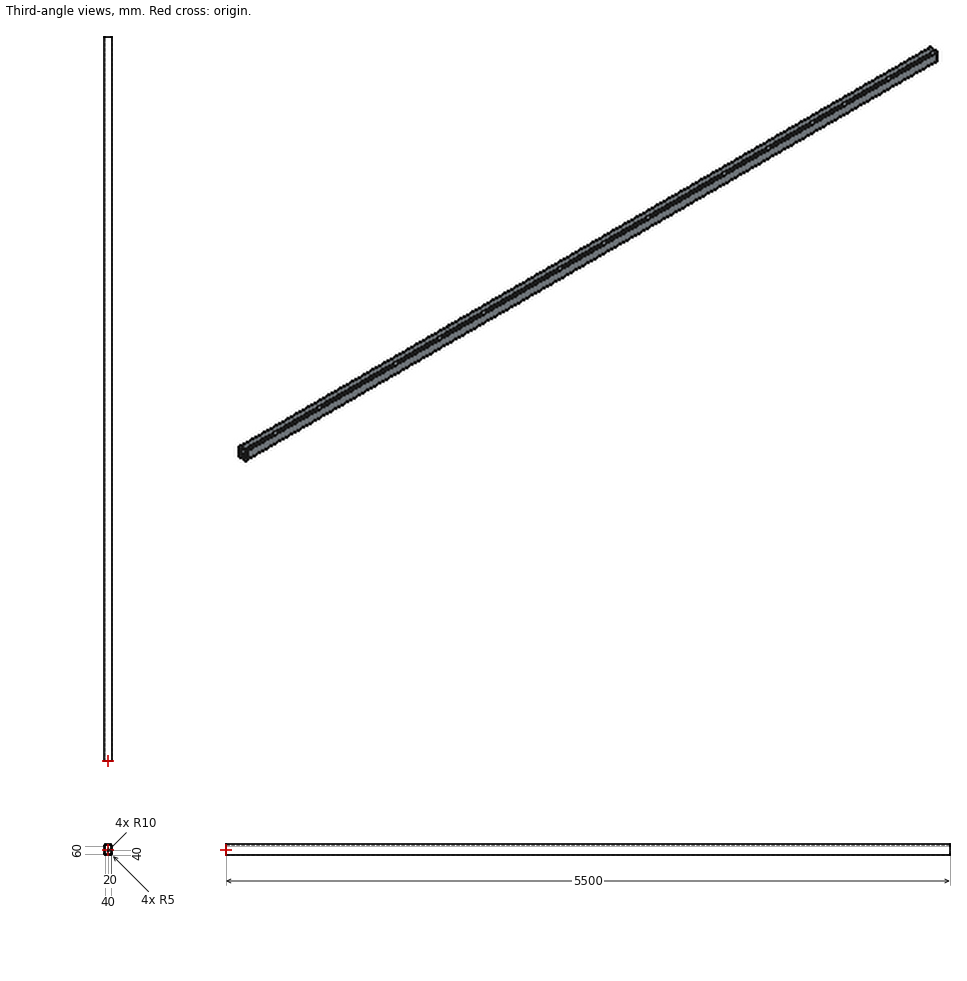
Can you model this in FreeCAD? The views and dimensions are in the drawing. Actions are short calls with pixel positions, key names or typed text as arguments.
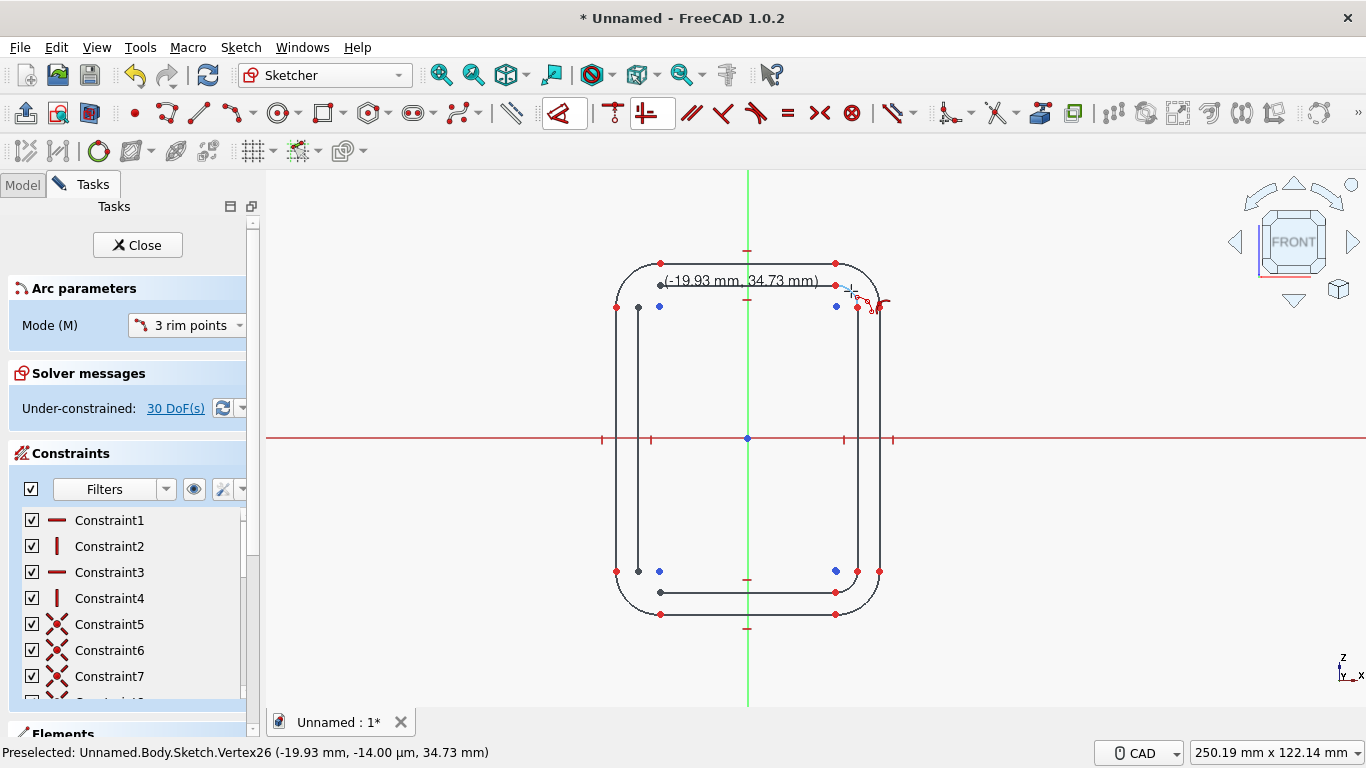
click(638, 307)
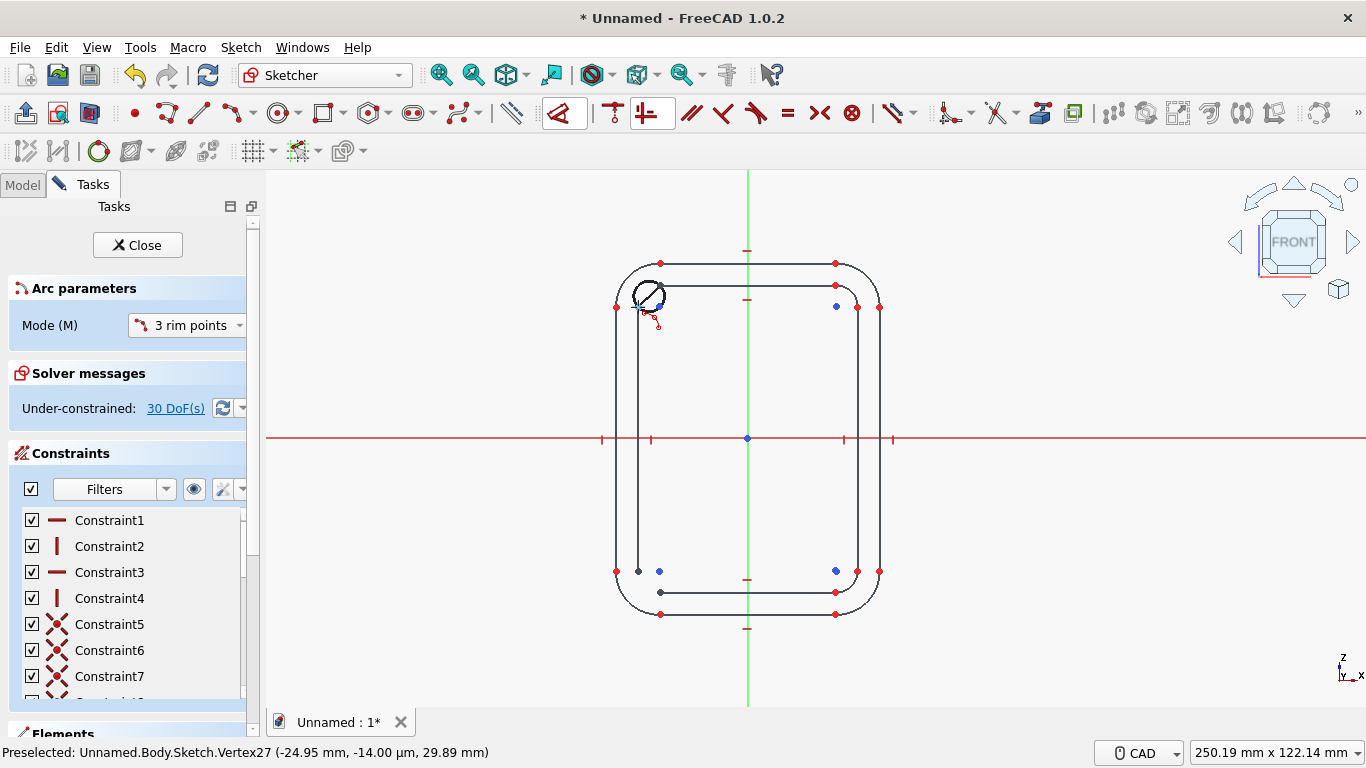
scroll(644, 291, up, 5)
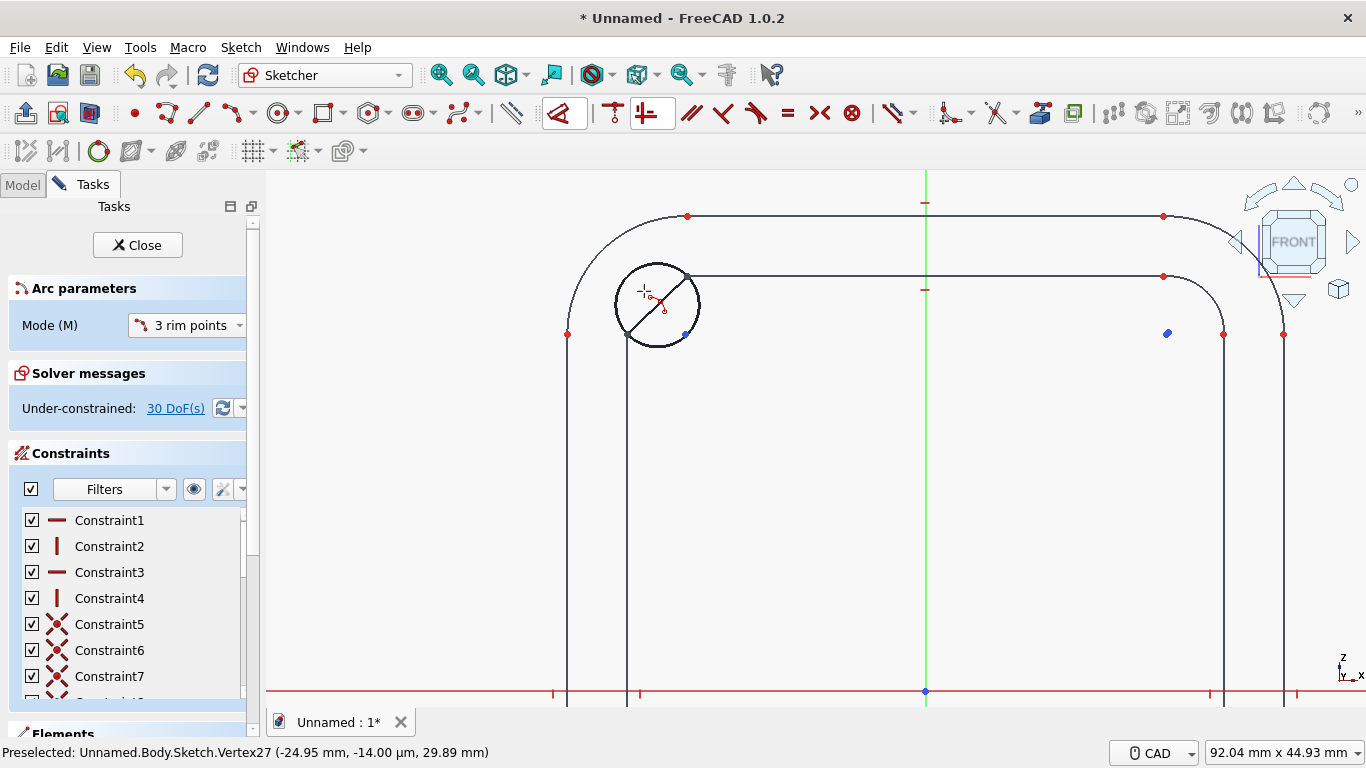
click(644, 291)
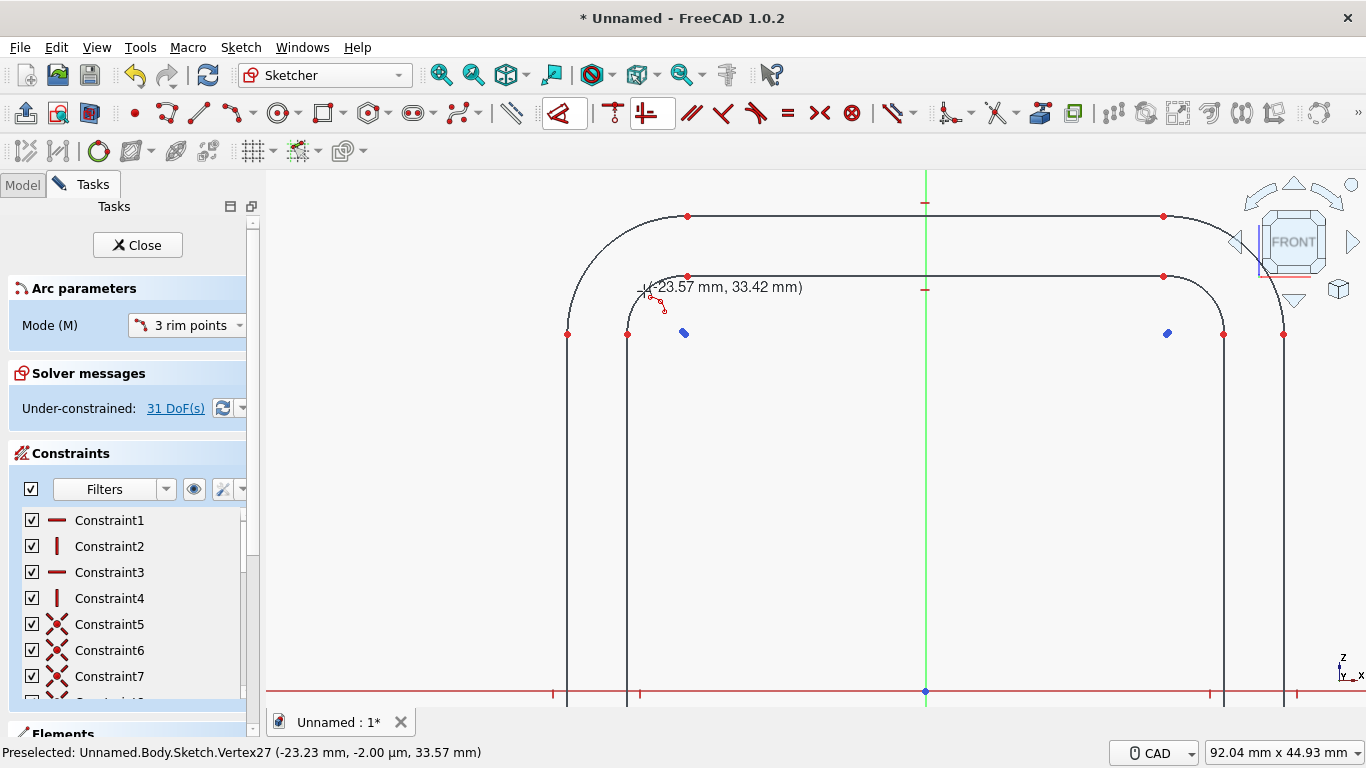
scroll(644, 291, down, 5)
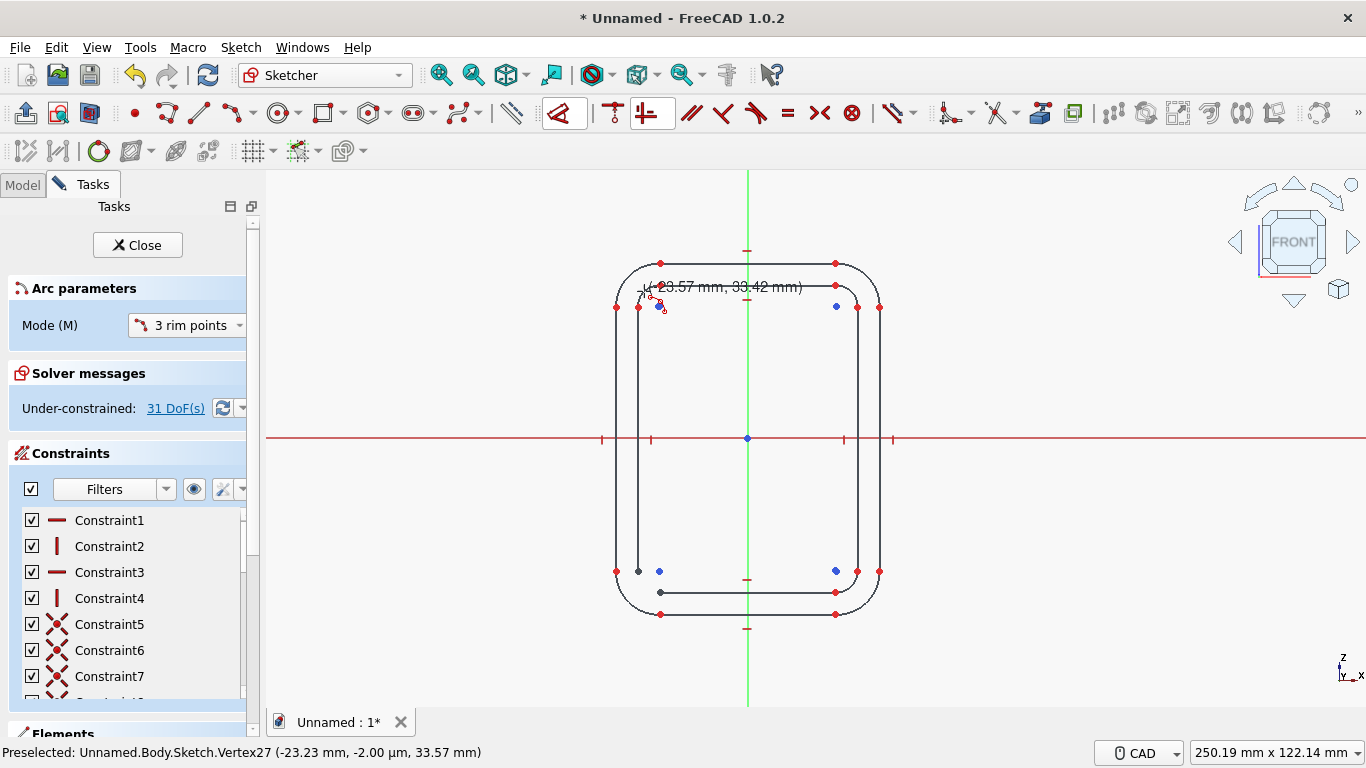
click(638, 571)
click(660, 593)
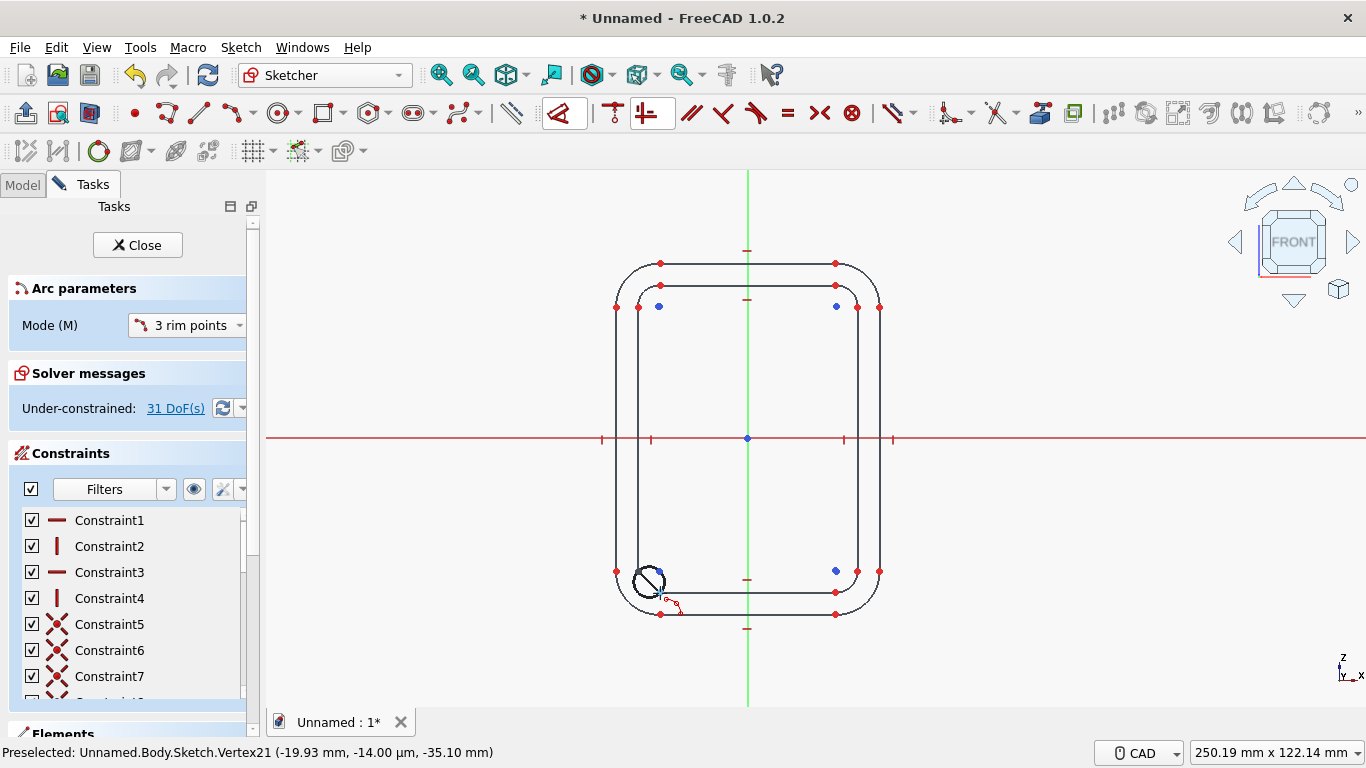
scroll(644, 586, up, 5)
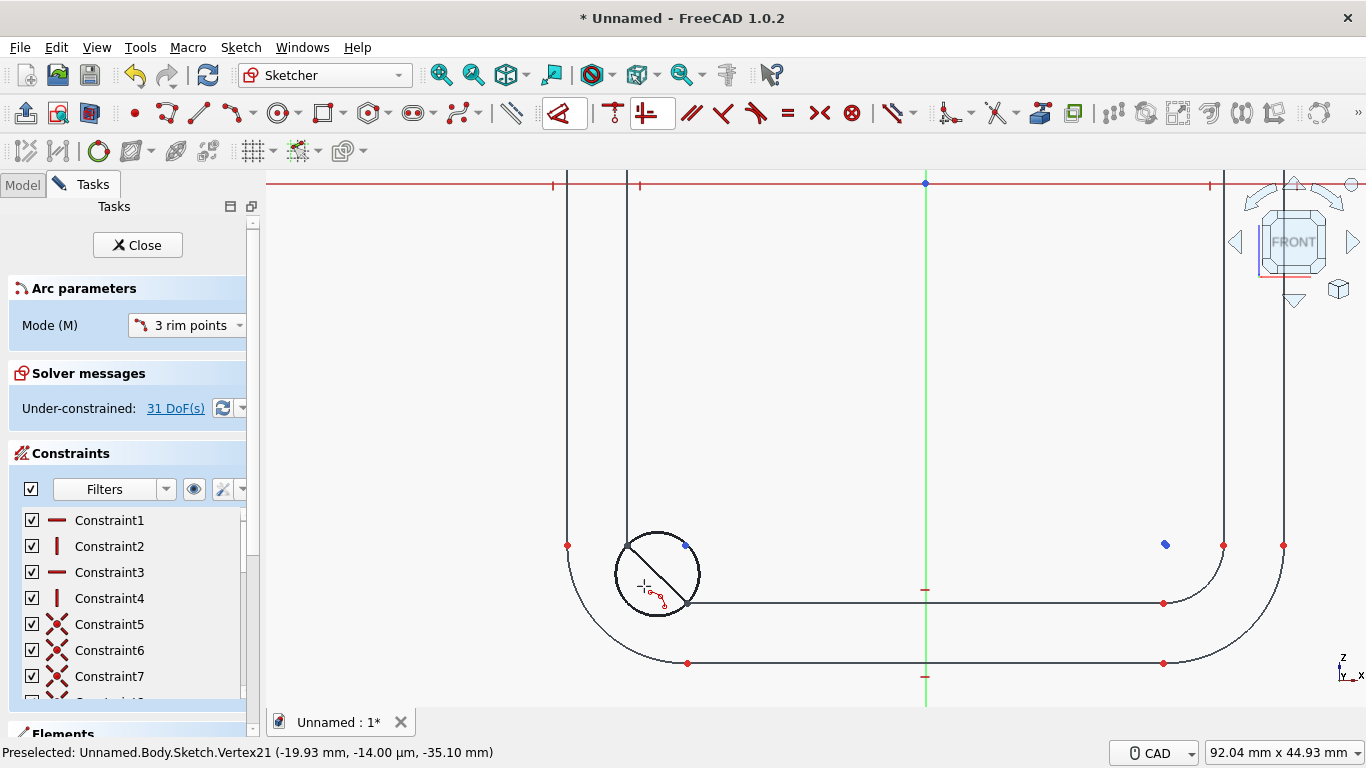
click(644, 584)
key(Escape)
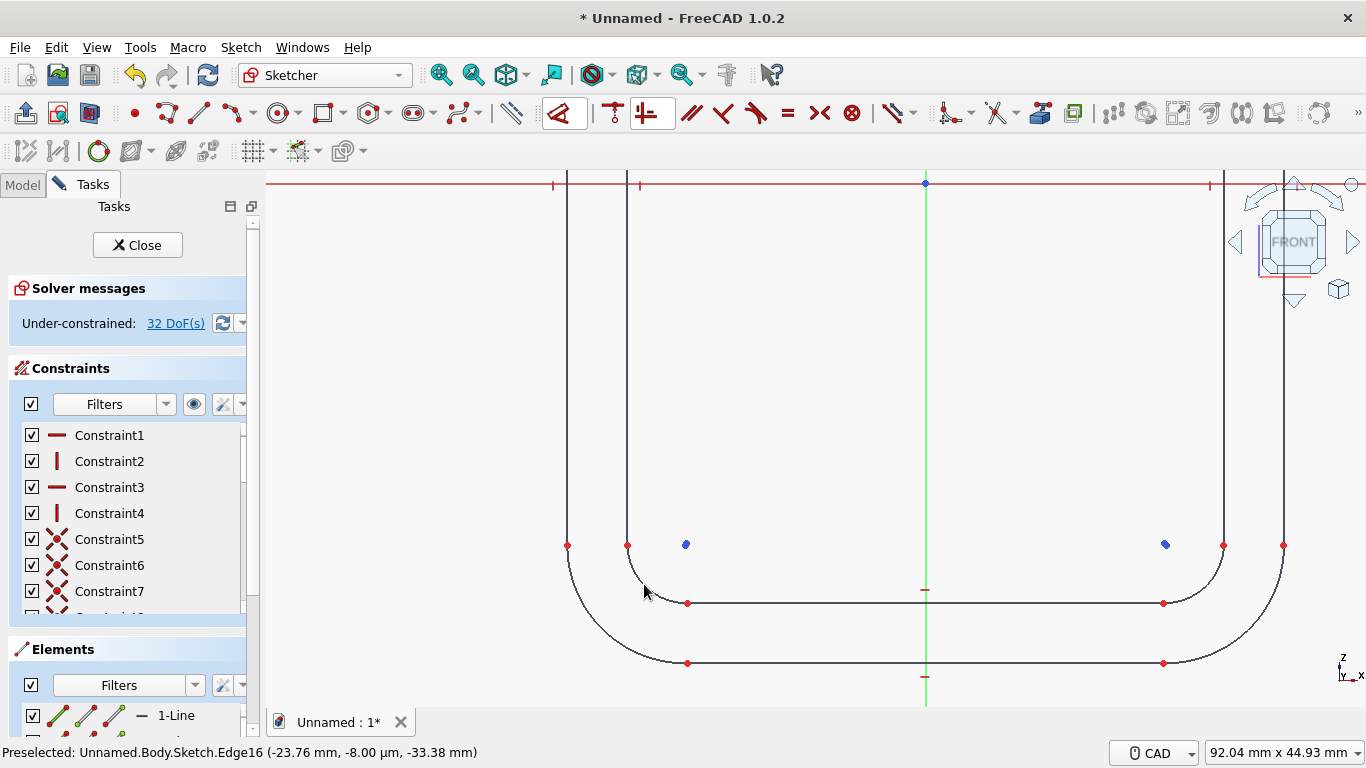
click(1021, 663)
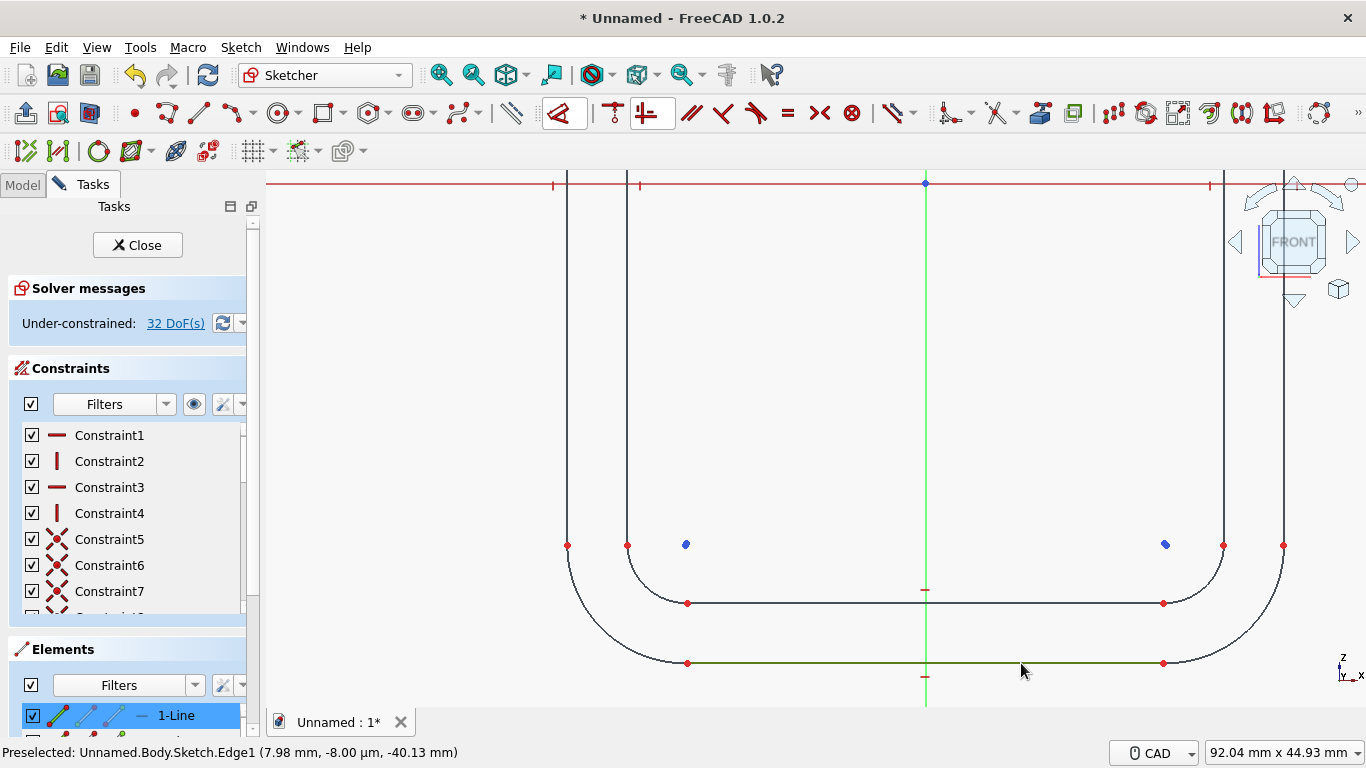
click(580, 599)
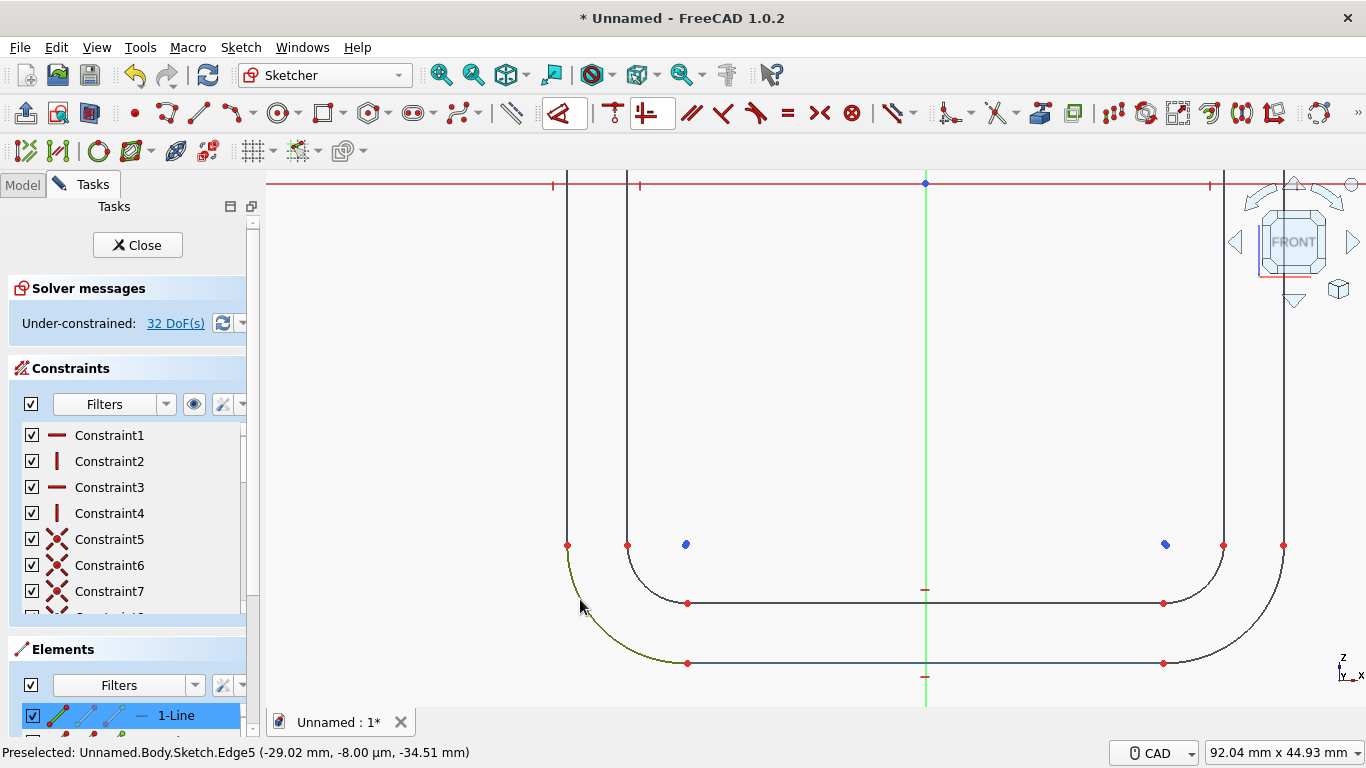
click(756, 114)